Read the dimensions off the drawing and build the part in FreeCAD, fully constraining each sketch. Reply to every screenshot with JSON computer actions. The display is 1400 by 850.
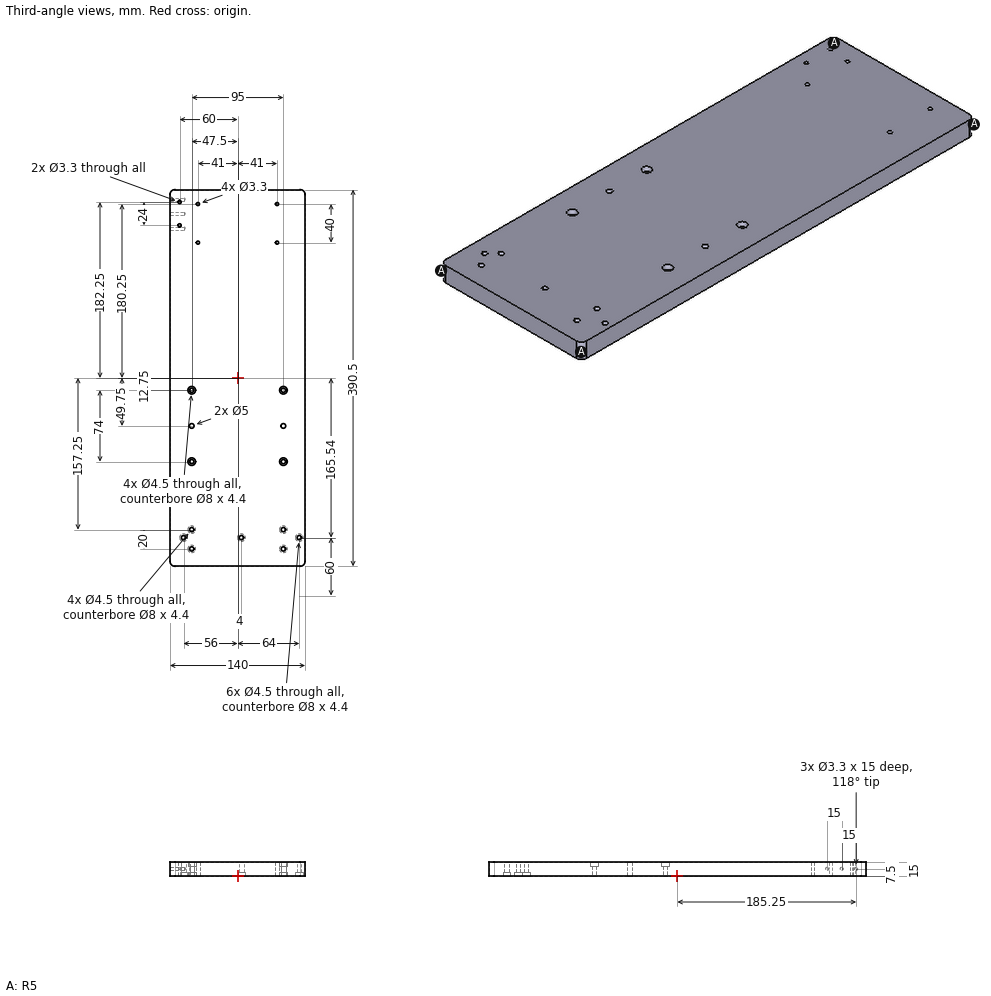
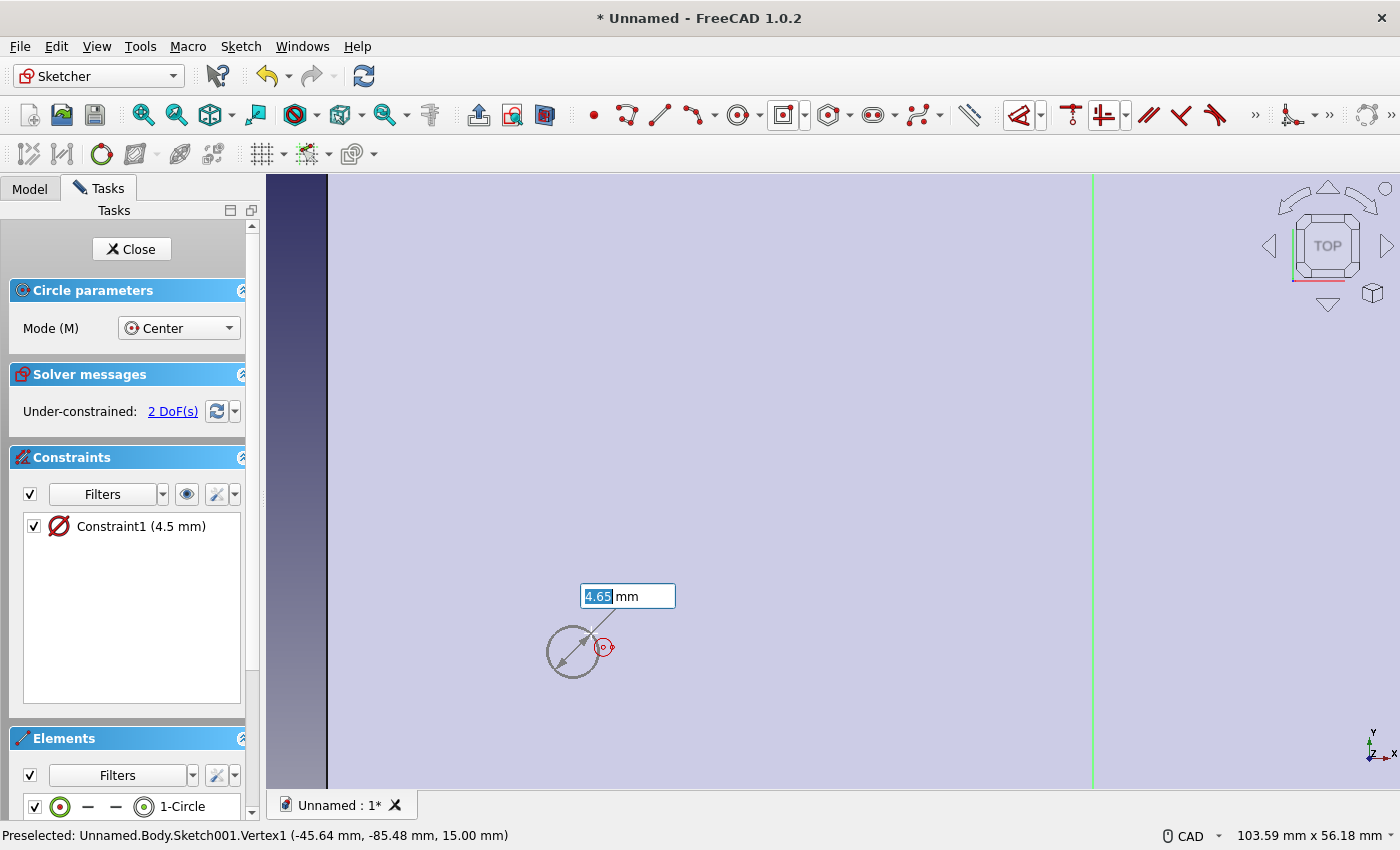
{"action": "type", "text": "4.5"}
{"action": "key", "text": "Return"}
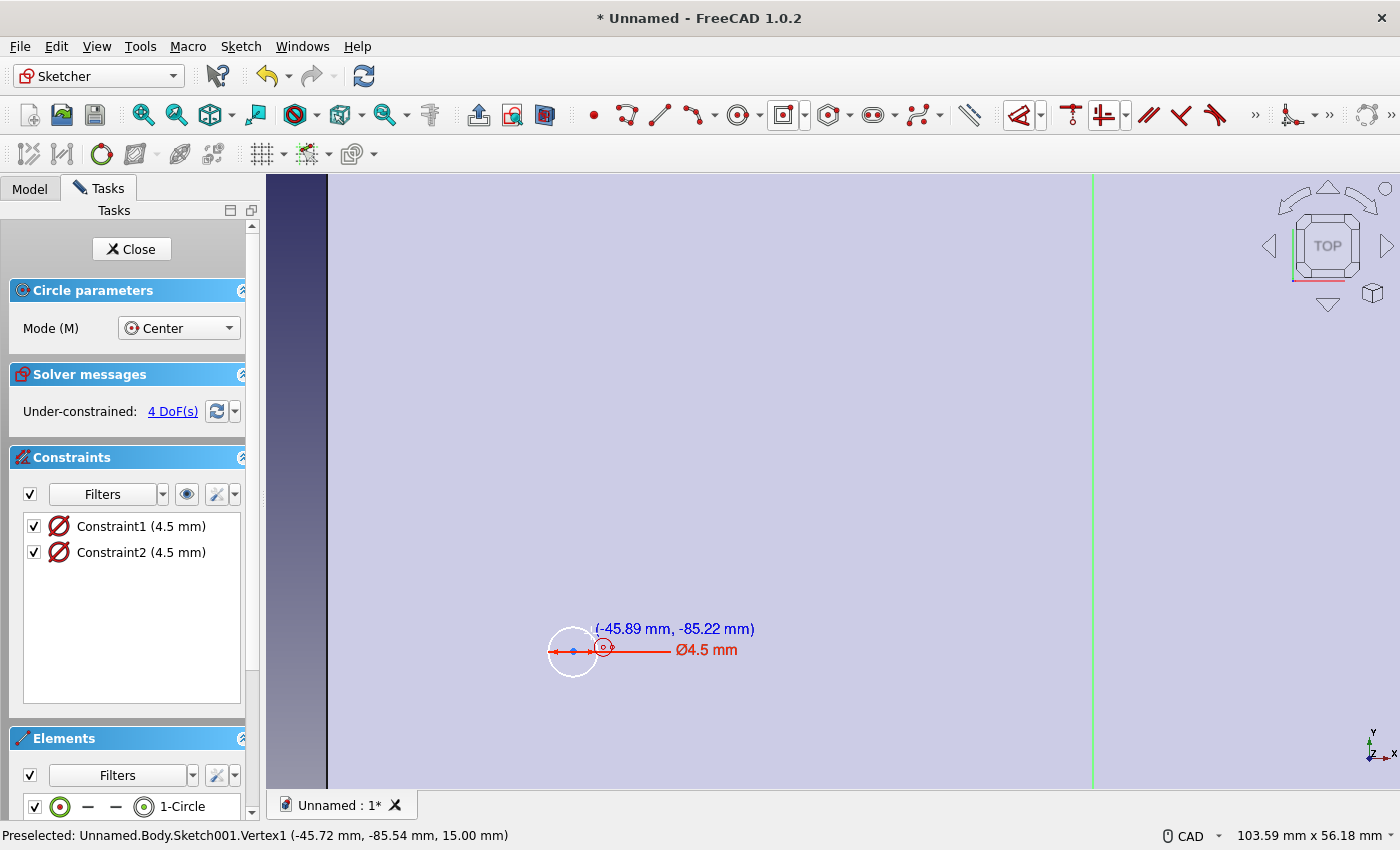
{"action": "scroll", "coordinate": [573, 652], "scroll_direction": "down", "scroll_amount": 5}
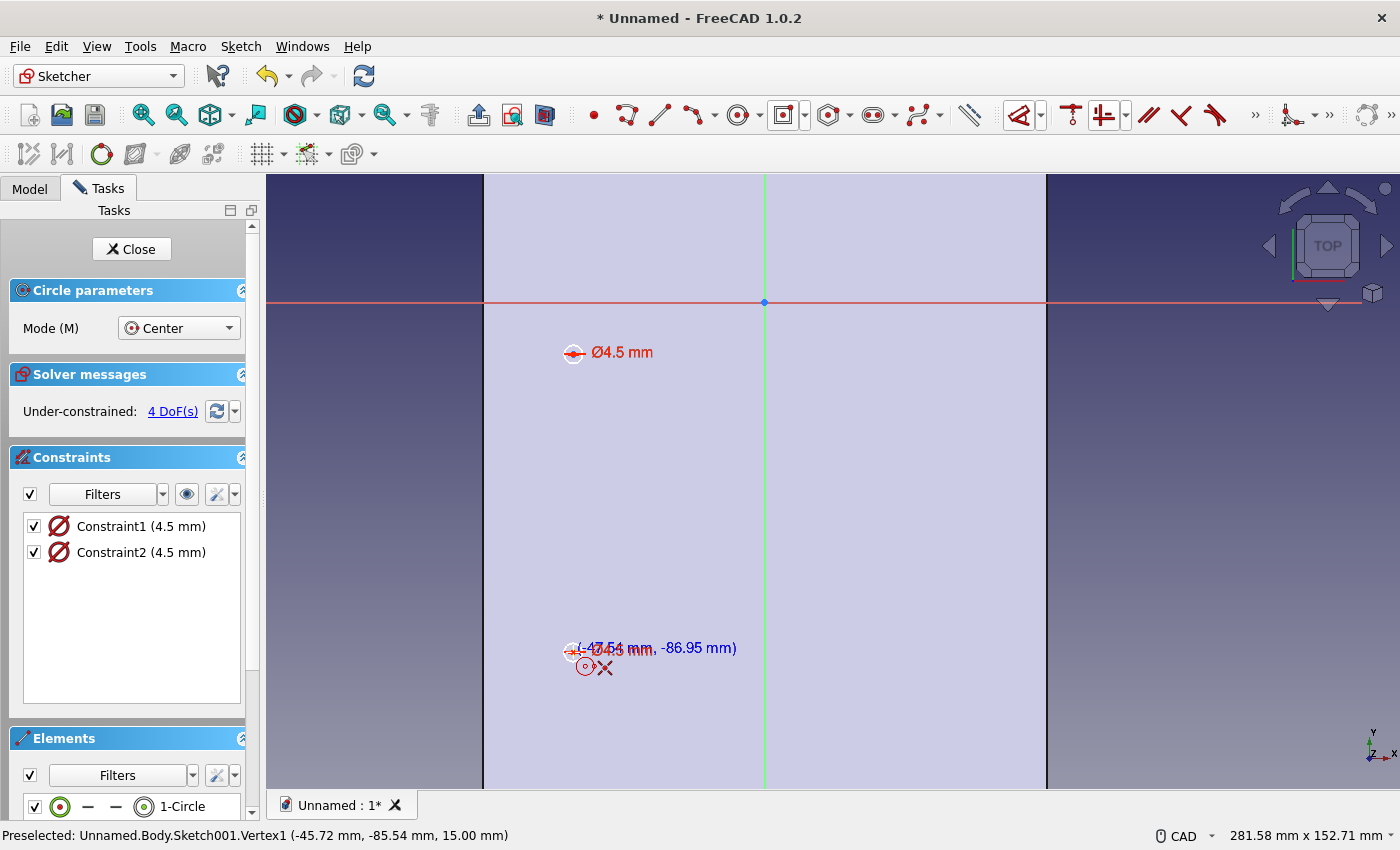
{"action": "scroll", "coordinate": [956, 354], "scroll_direction": "up", "scroll_amount": 5}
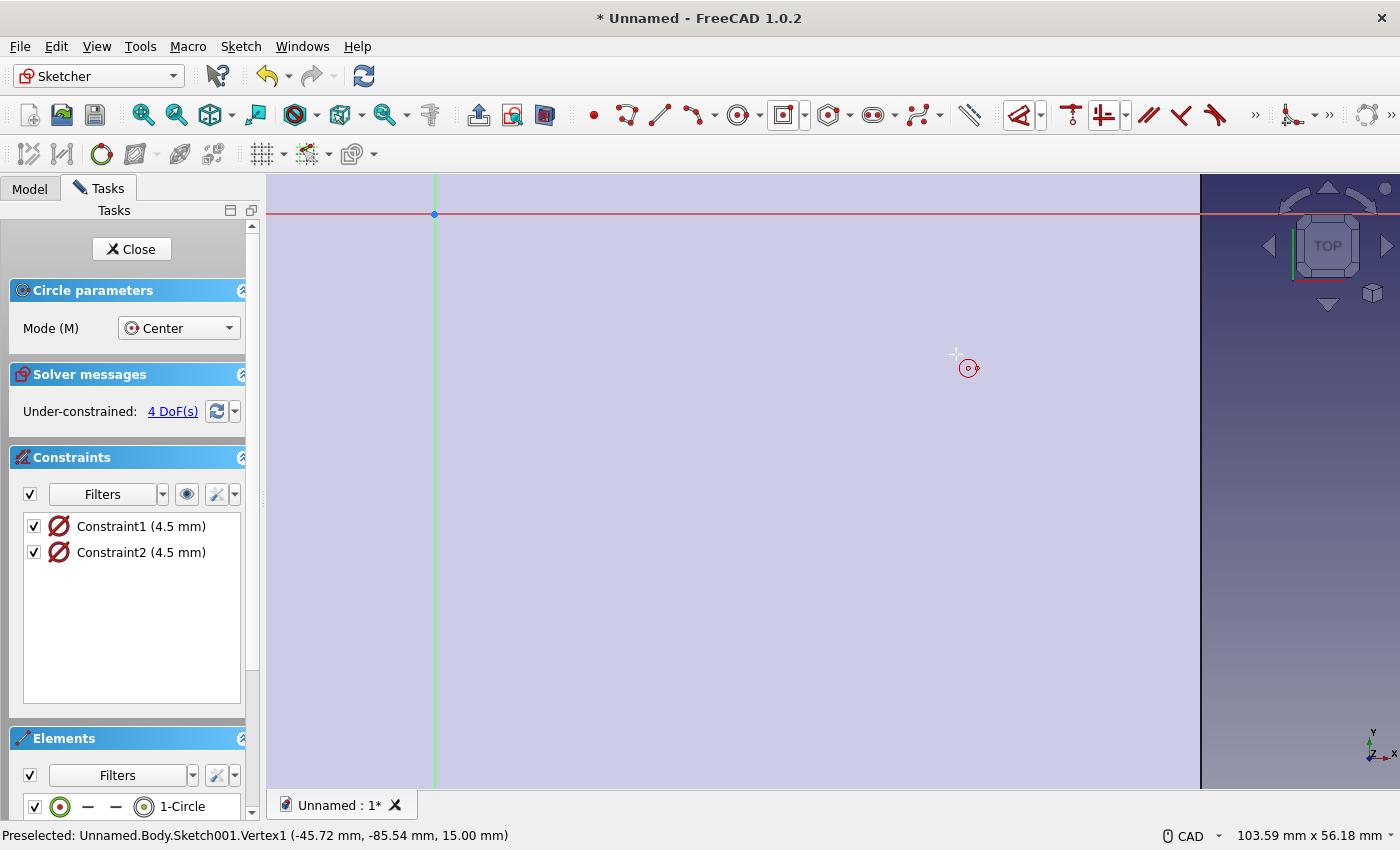
{"action": "left_click", "coordinate": [955, 354]}
{"action": "mouse_move", "coordinate": [972, 336]}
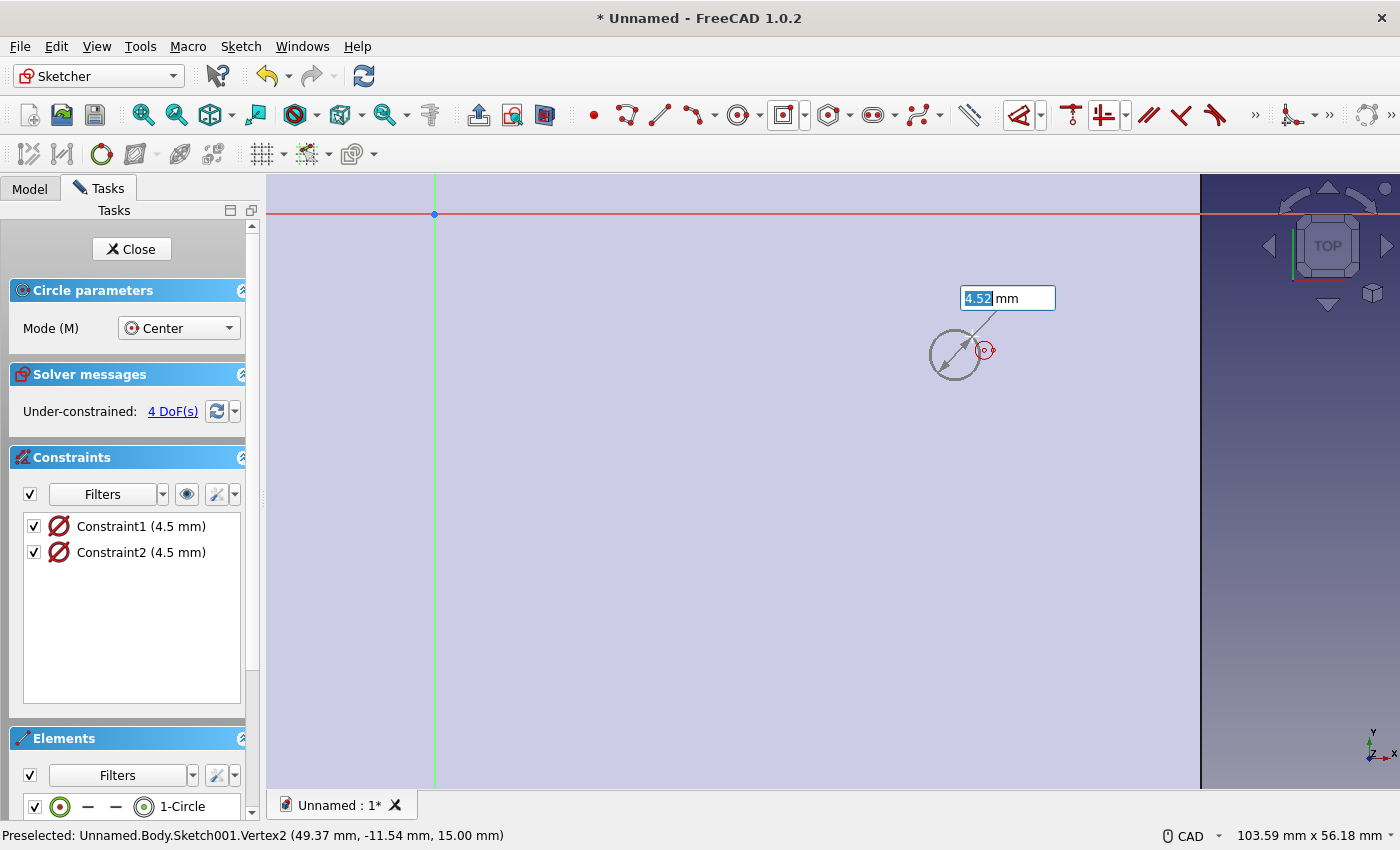
{"action": "type", "text": "4.5"}
{"action": "key", "text": "Return"}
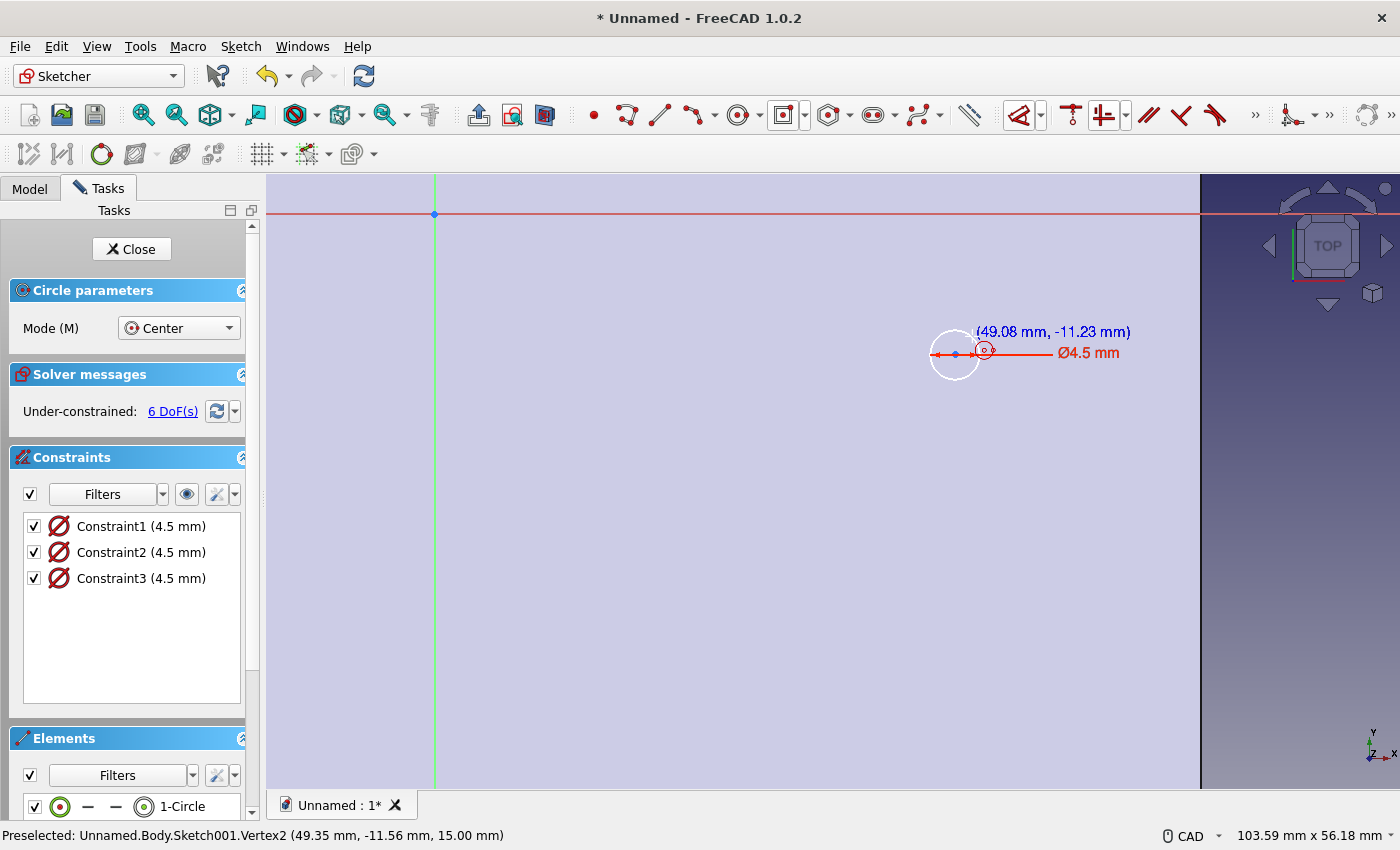
{"action": "scroll", "coordinate": [956, 354], "scroll_direction": "down", "scroll_amount": 5}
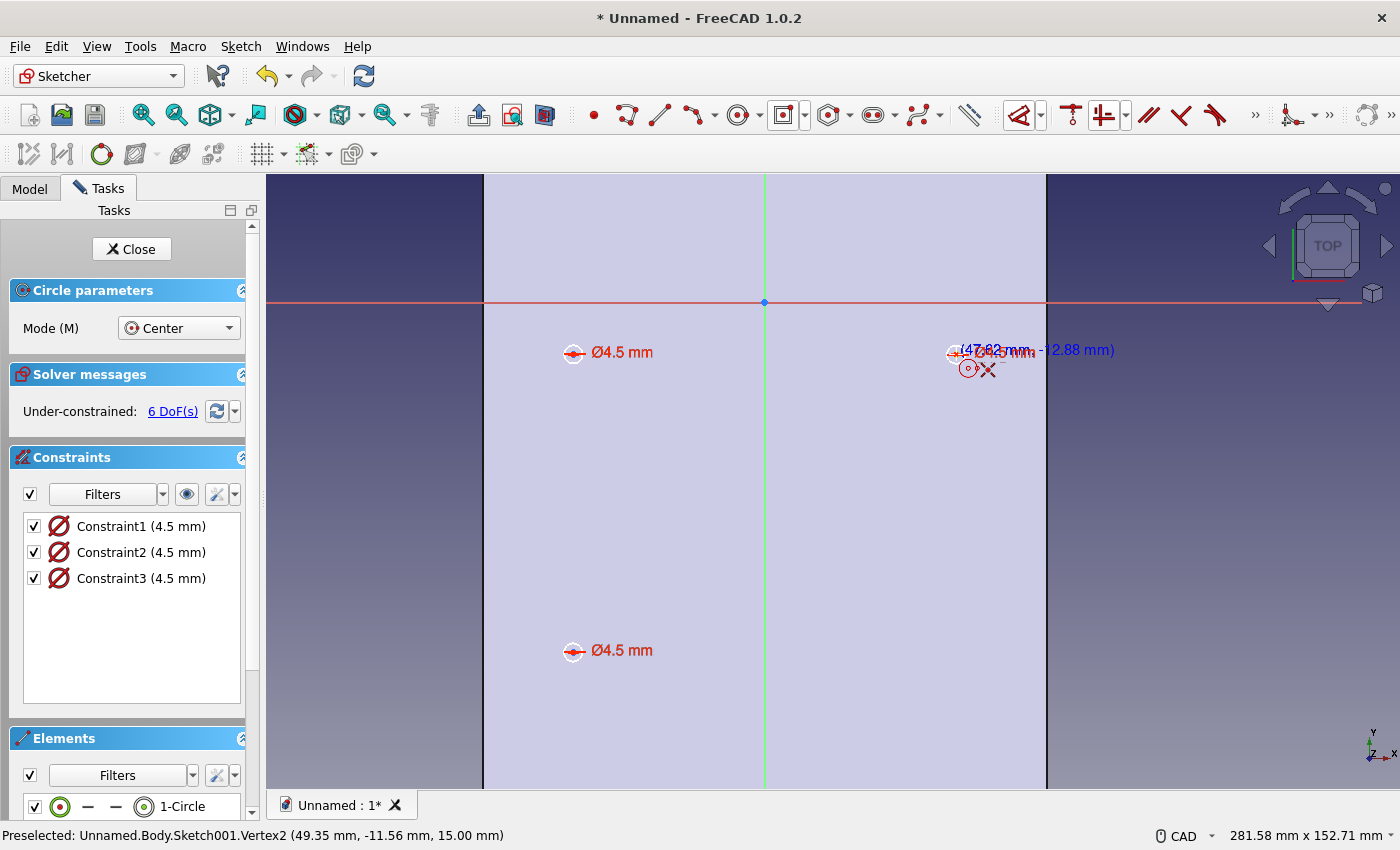
{"action": "scroll", "coordinate": [956, 652], "scroll_direction": "up", "scroll_amount": 5}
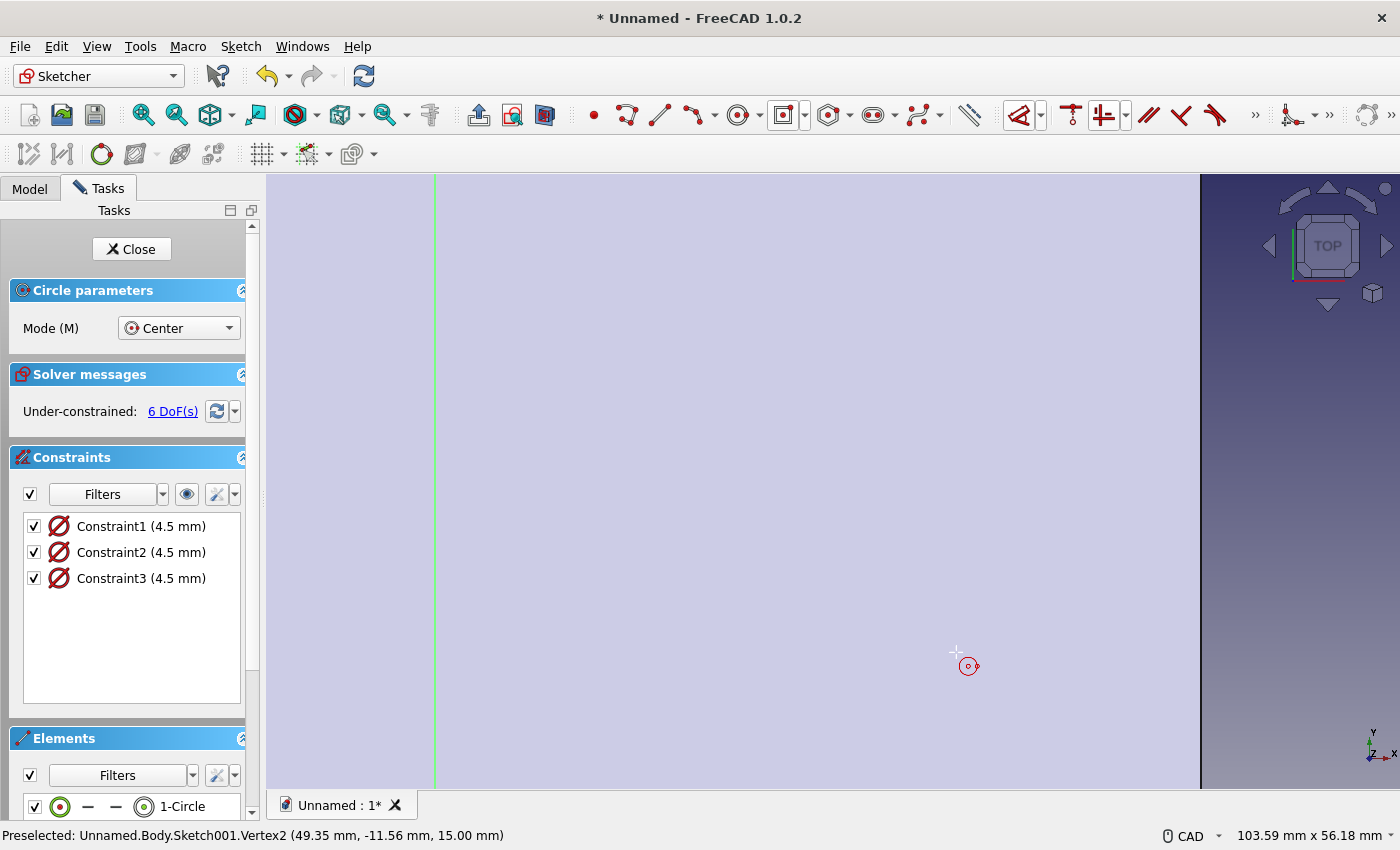
{"action": "left_click", "coordinate": [955, 651]}
{"action": "mouse_move", "coordinate": [972, 633]}